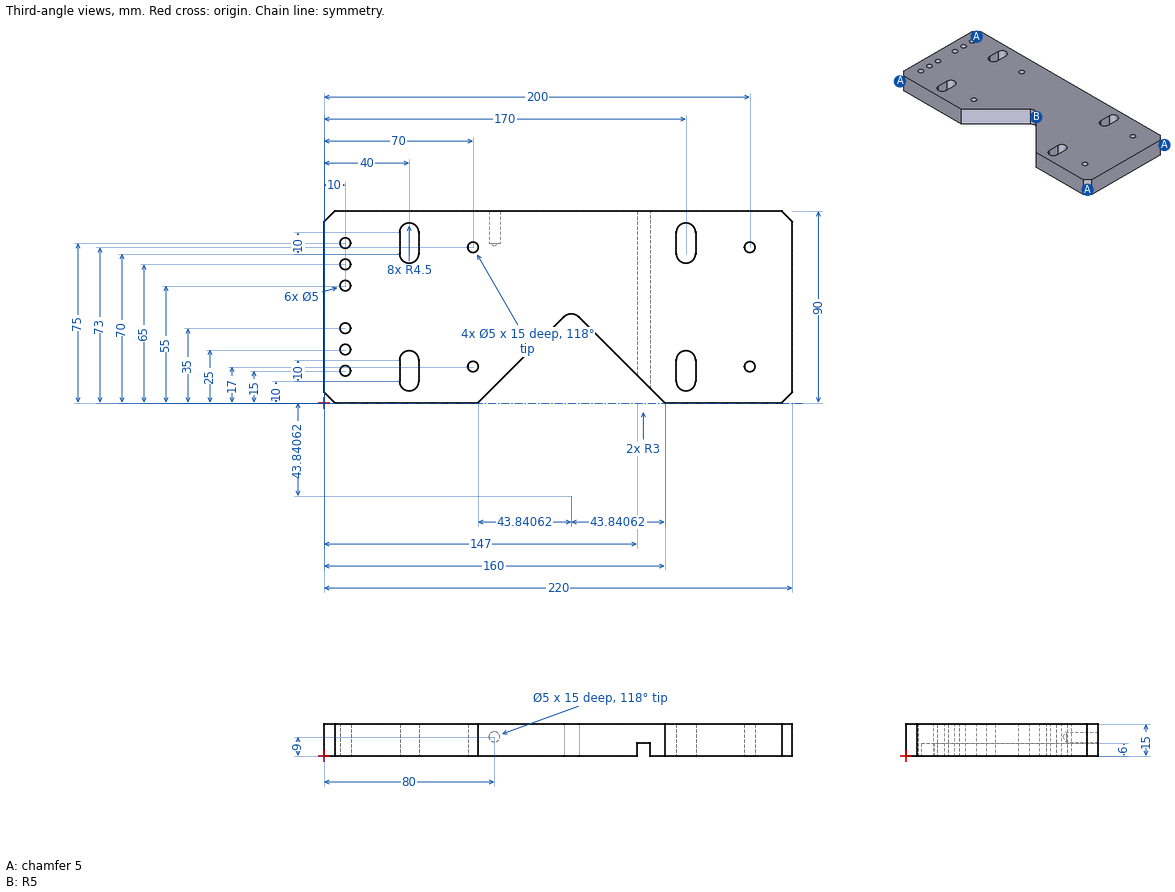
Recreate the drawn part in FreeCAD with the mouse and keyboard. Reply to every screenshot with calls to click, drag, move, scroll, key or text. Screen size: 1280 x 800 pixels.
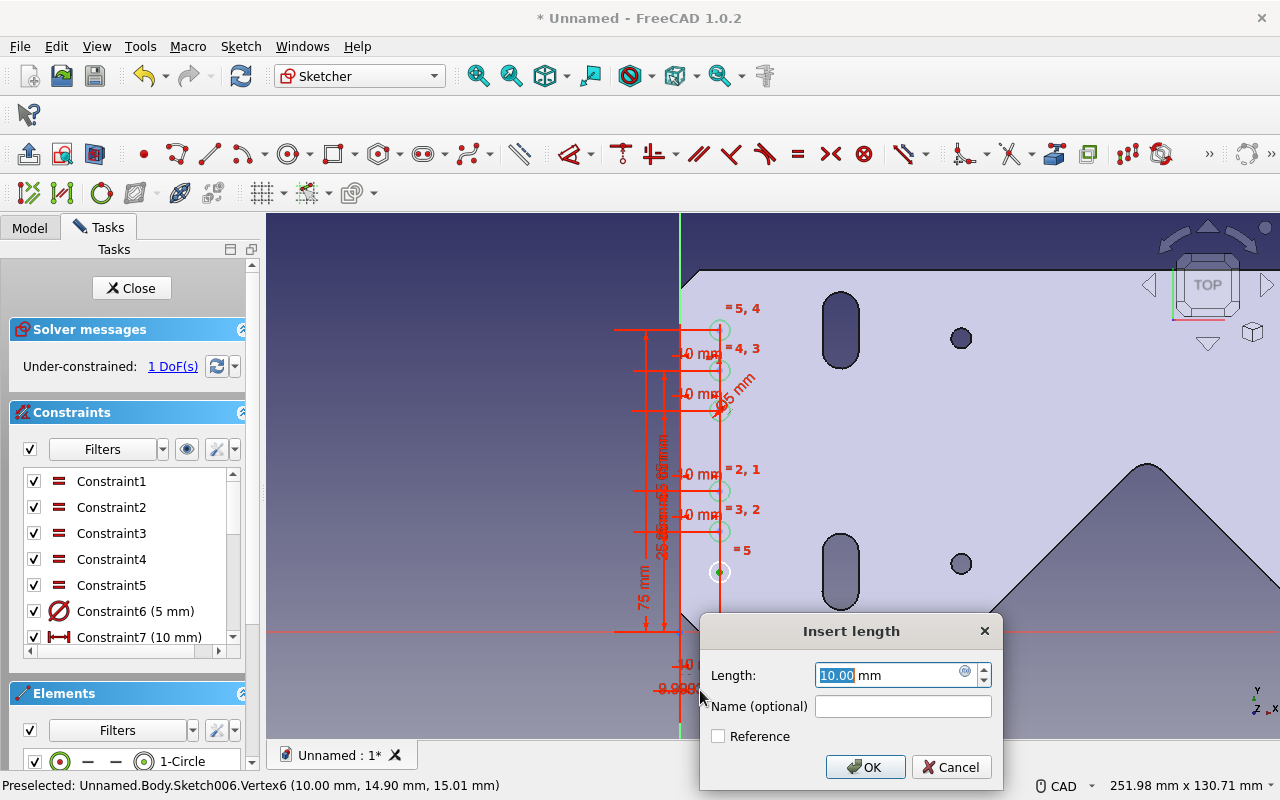
text(10)
key(Return)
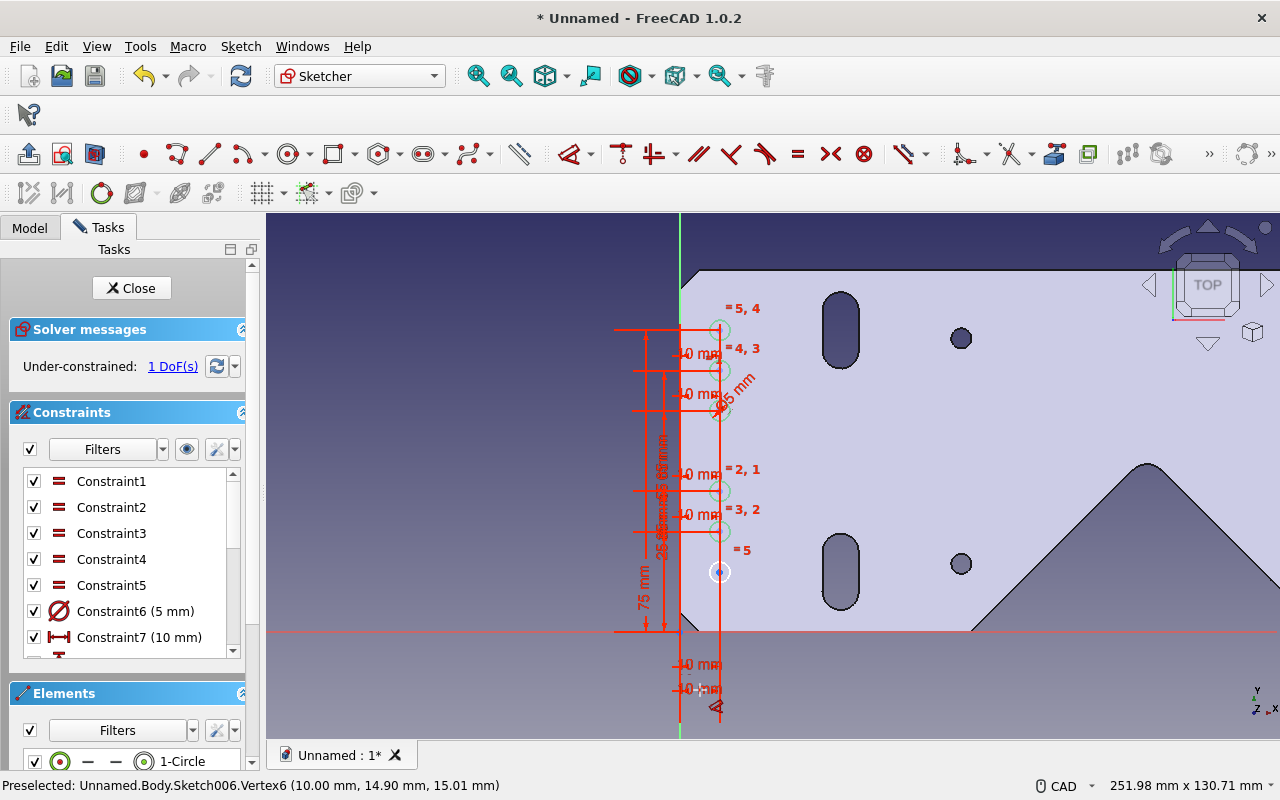
click(720, 572)
click(646, 616)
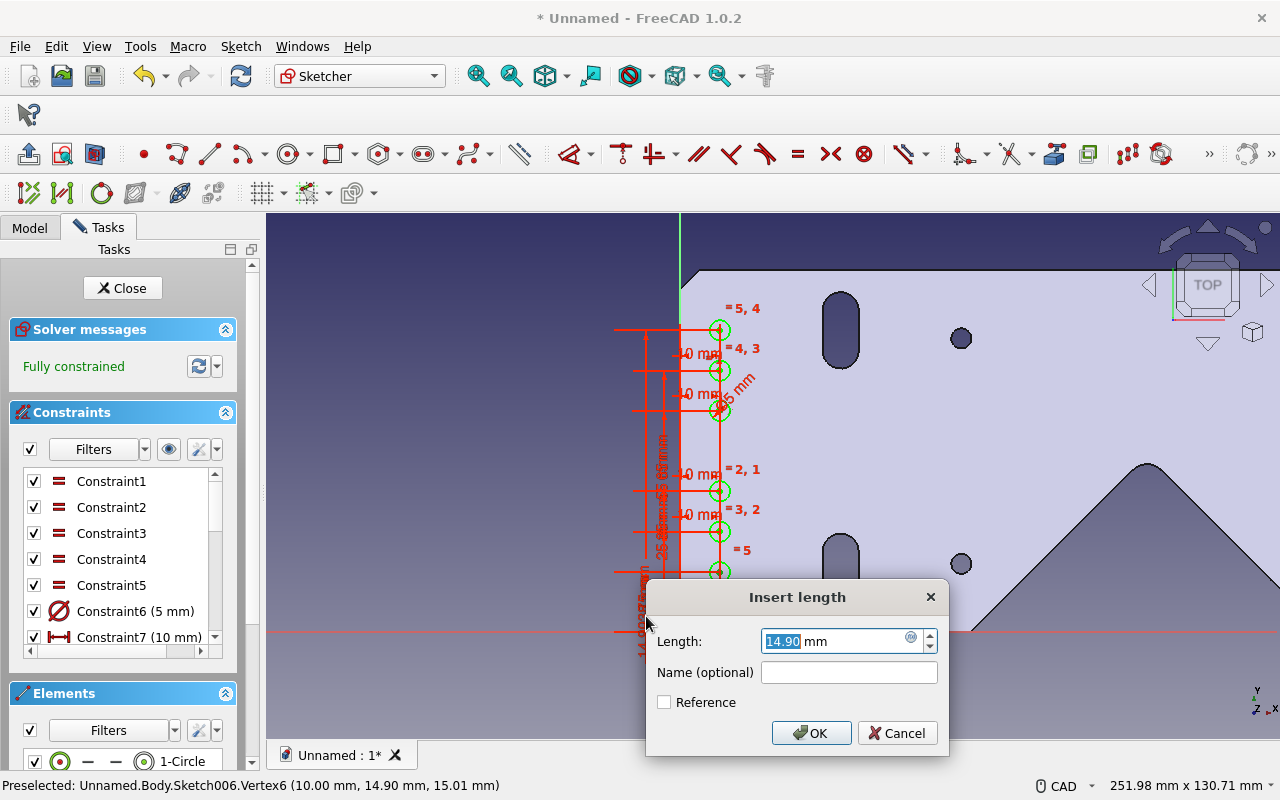
text(15)
key(Return)
key(Escape)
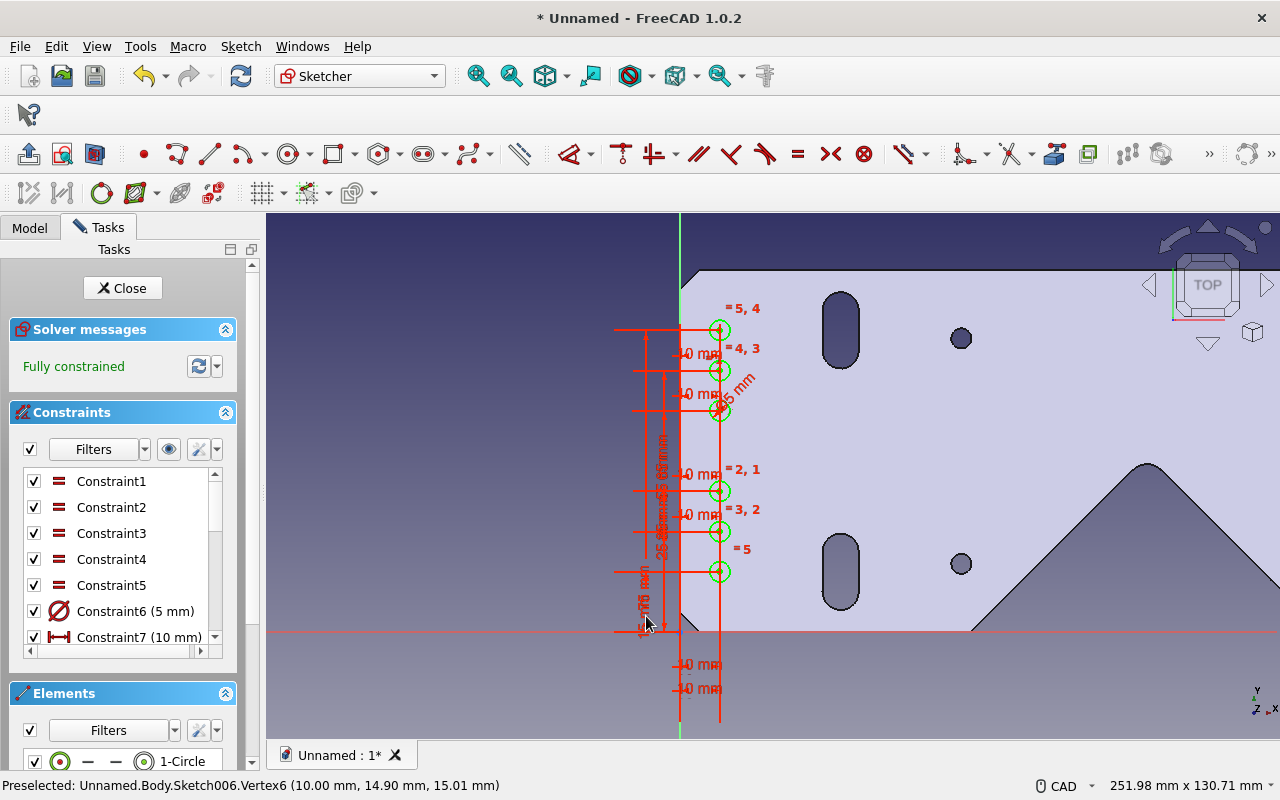
click(123, 288)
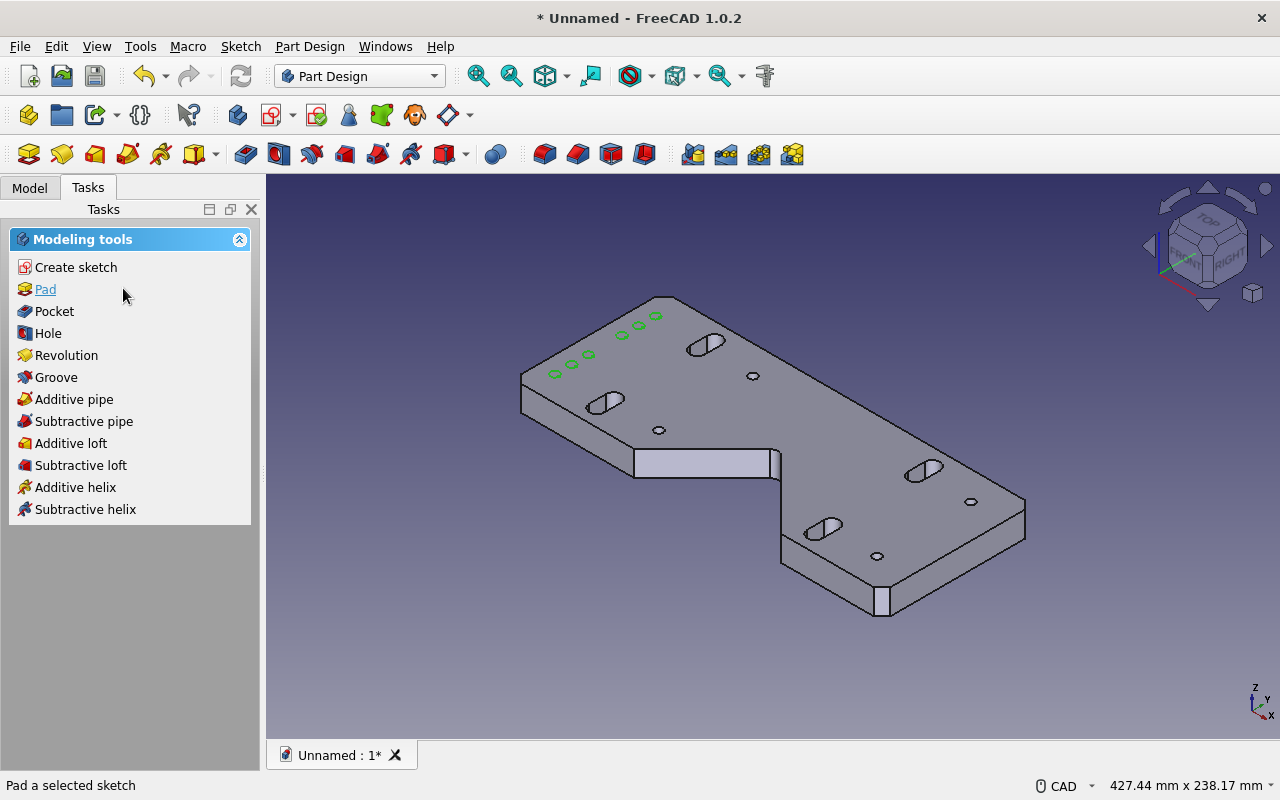
click(246, 154)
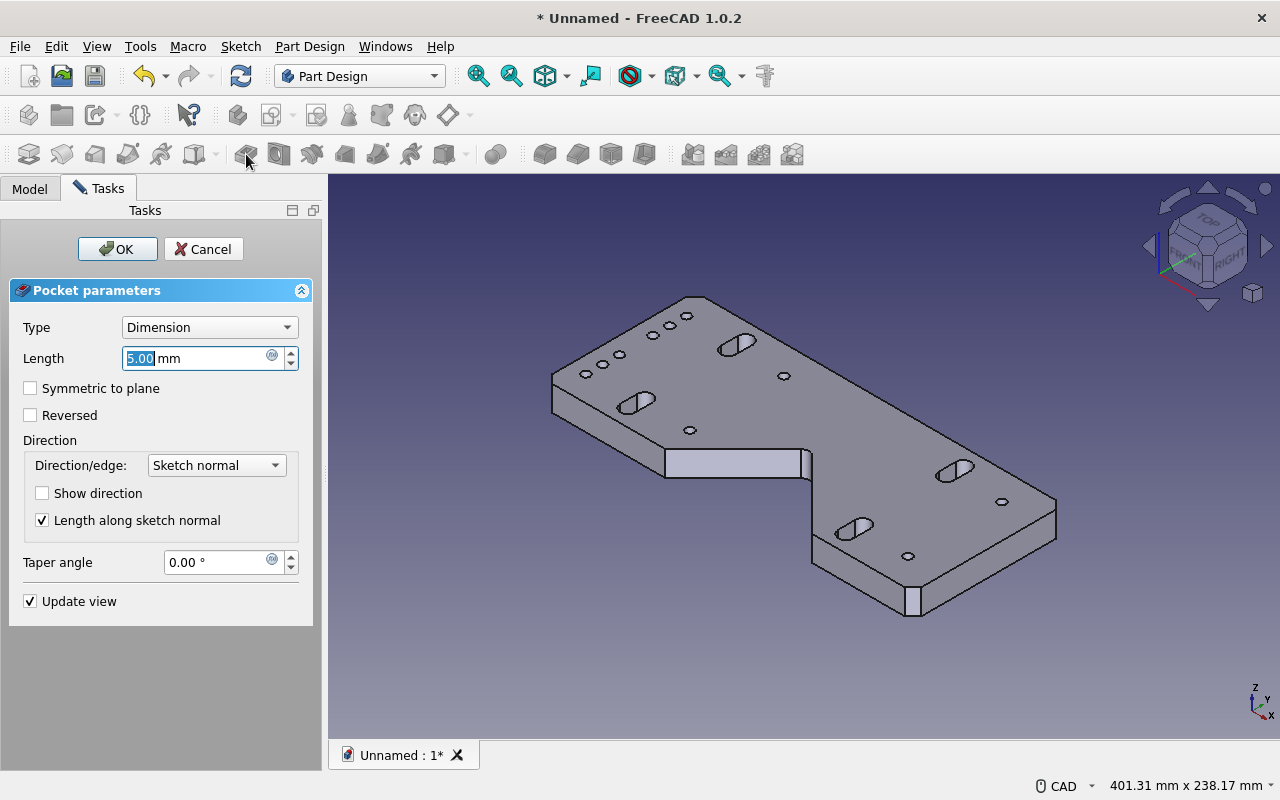
click(210, 328)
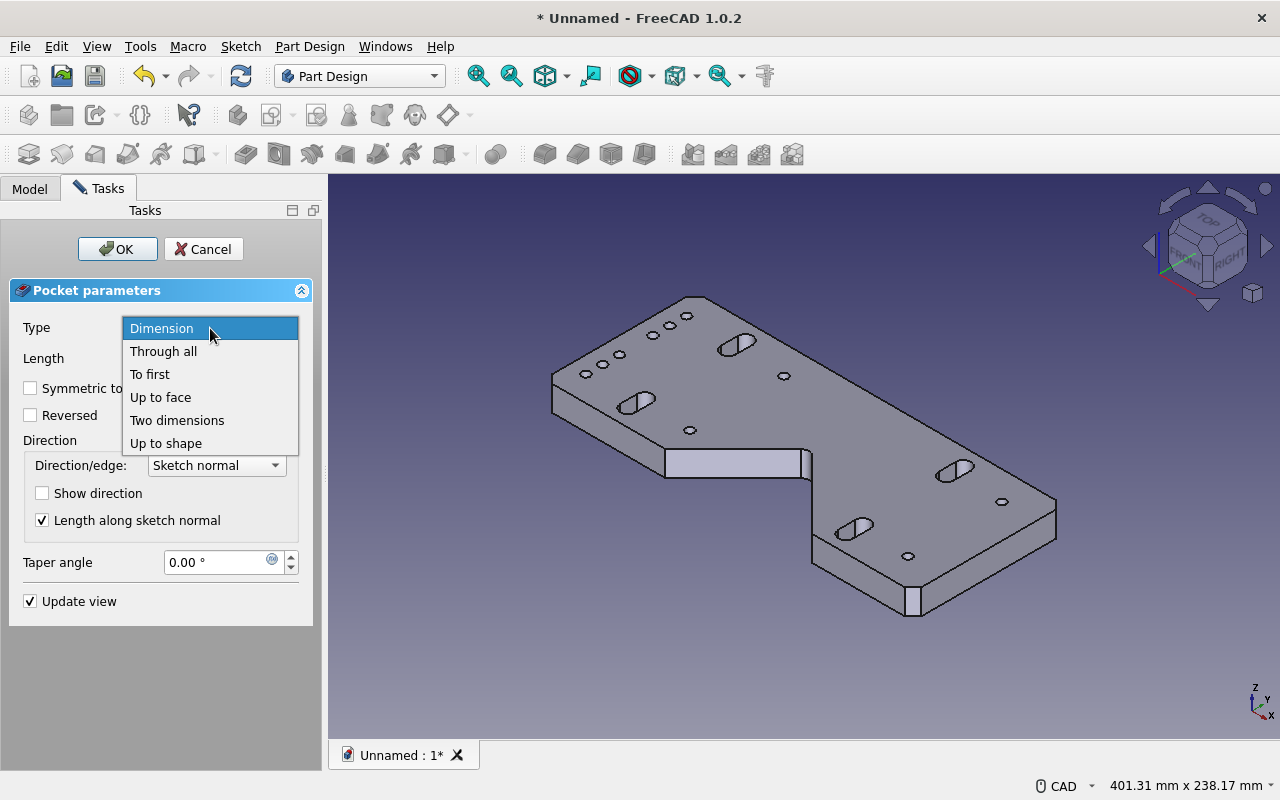
click(208, 352)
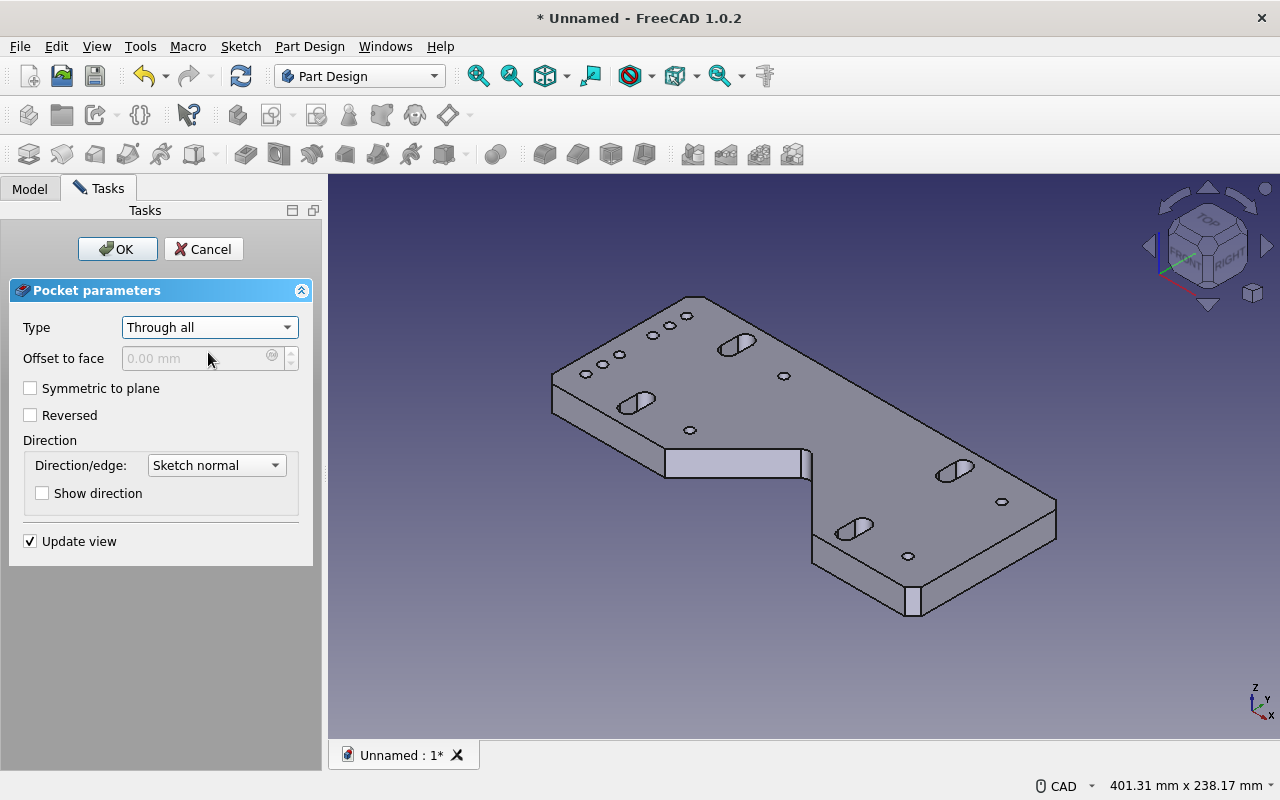
click(118, 249)